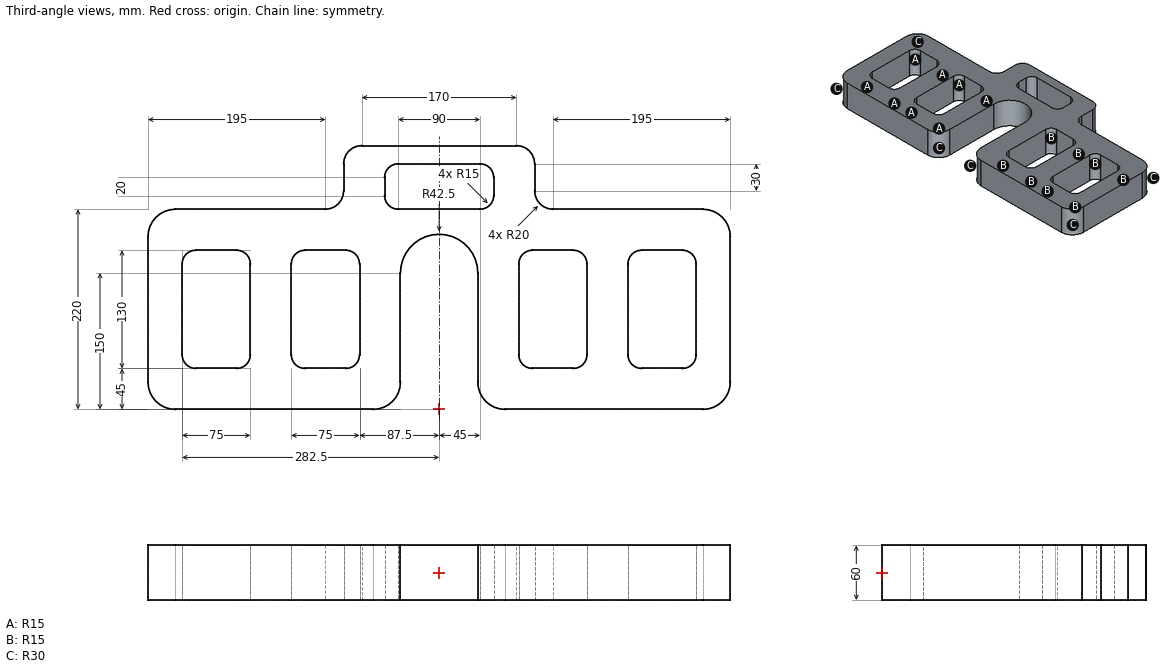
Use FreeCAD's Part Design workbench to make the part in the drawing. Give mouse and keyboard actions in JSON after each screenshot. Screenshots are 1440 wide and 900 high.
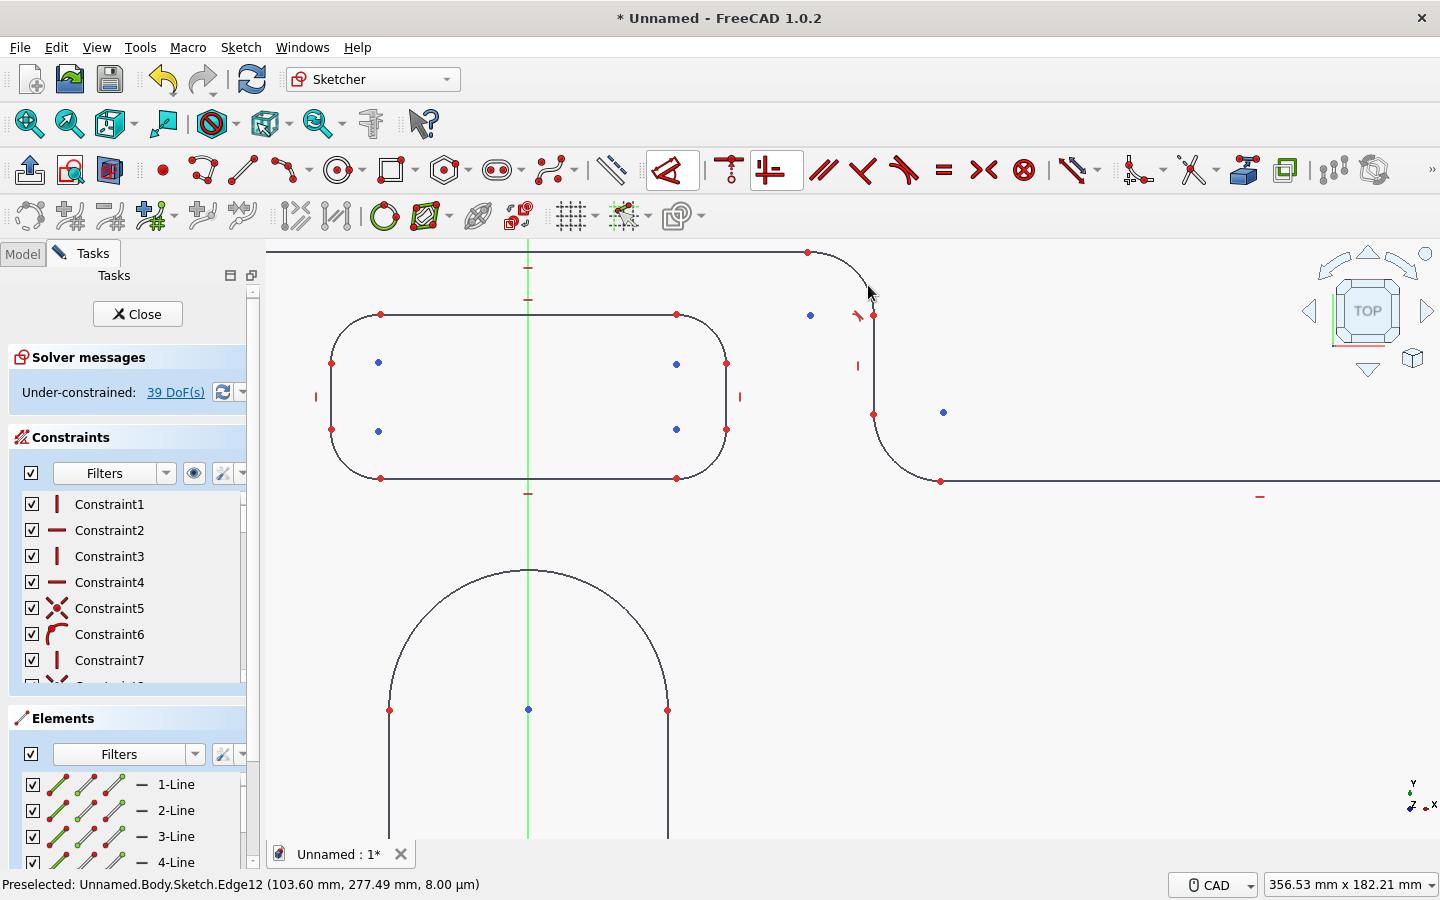
{"action": "left_click", "coordinate": [874, 385]}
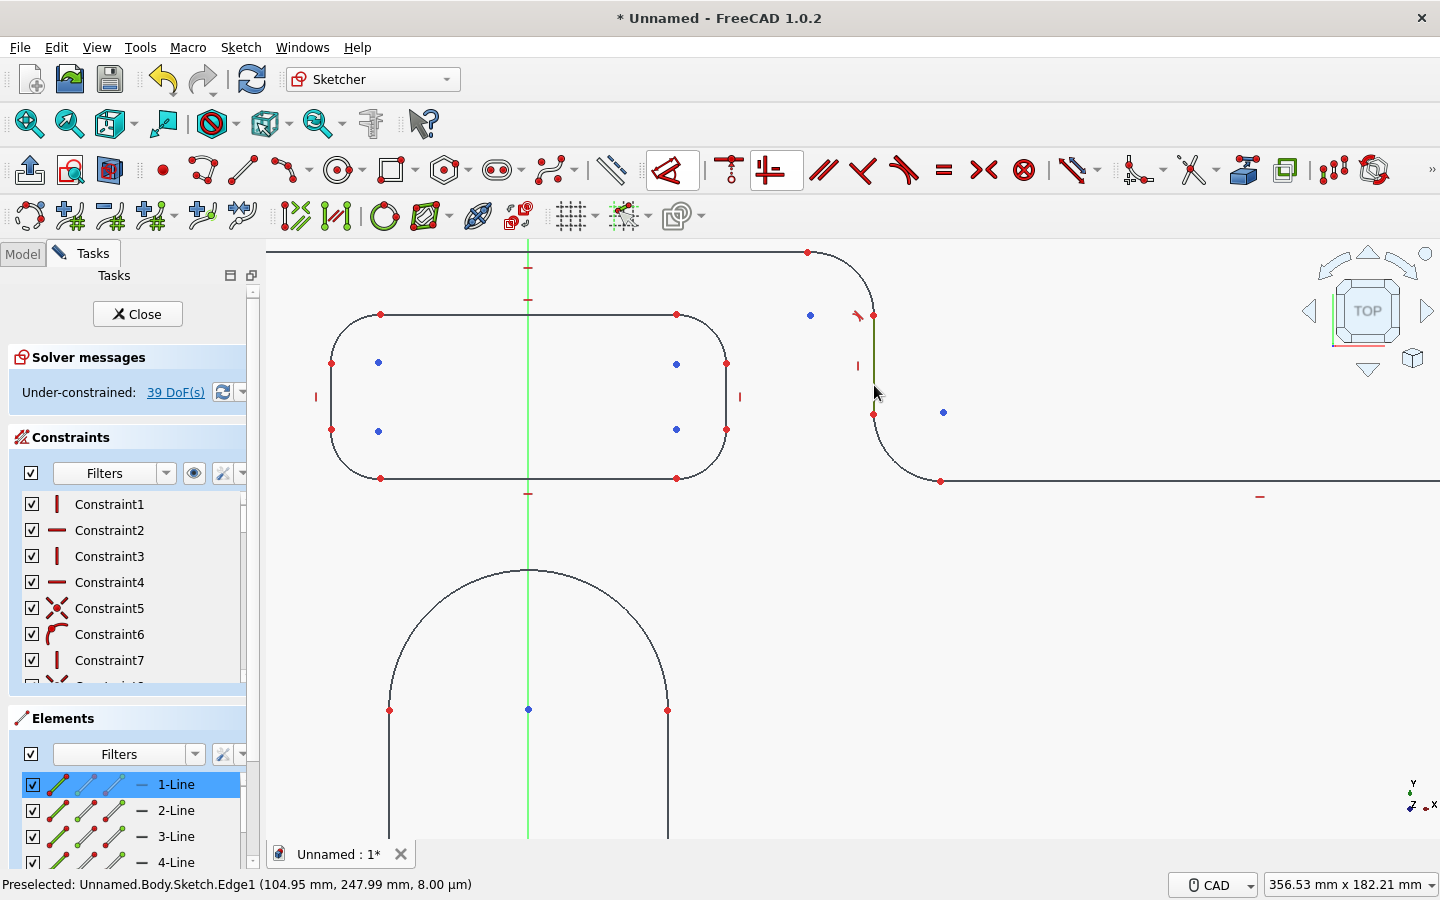
{"action": "left_click", "coordinate": [882, 445]}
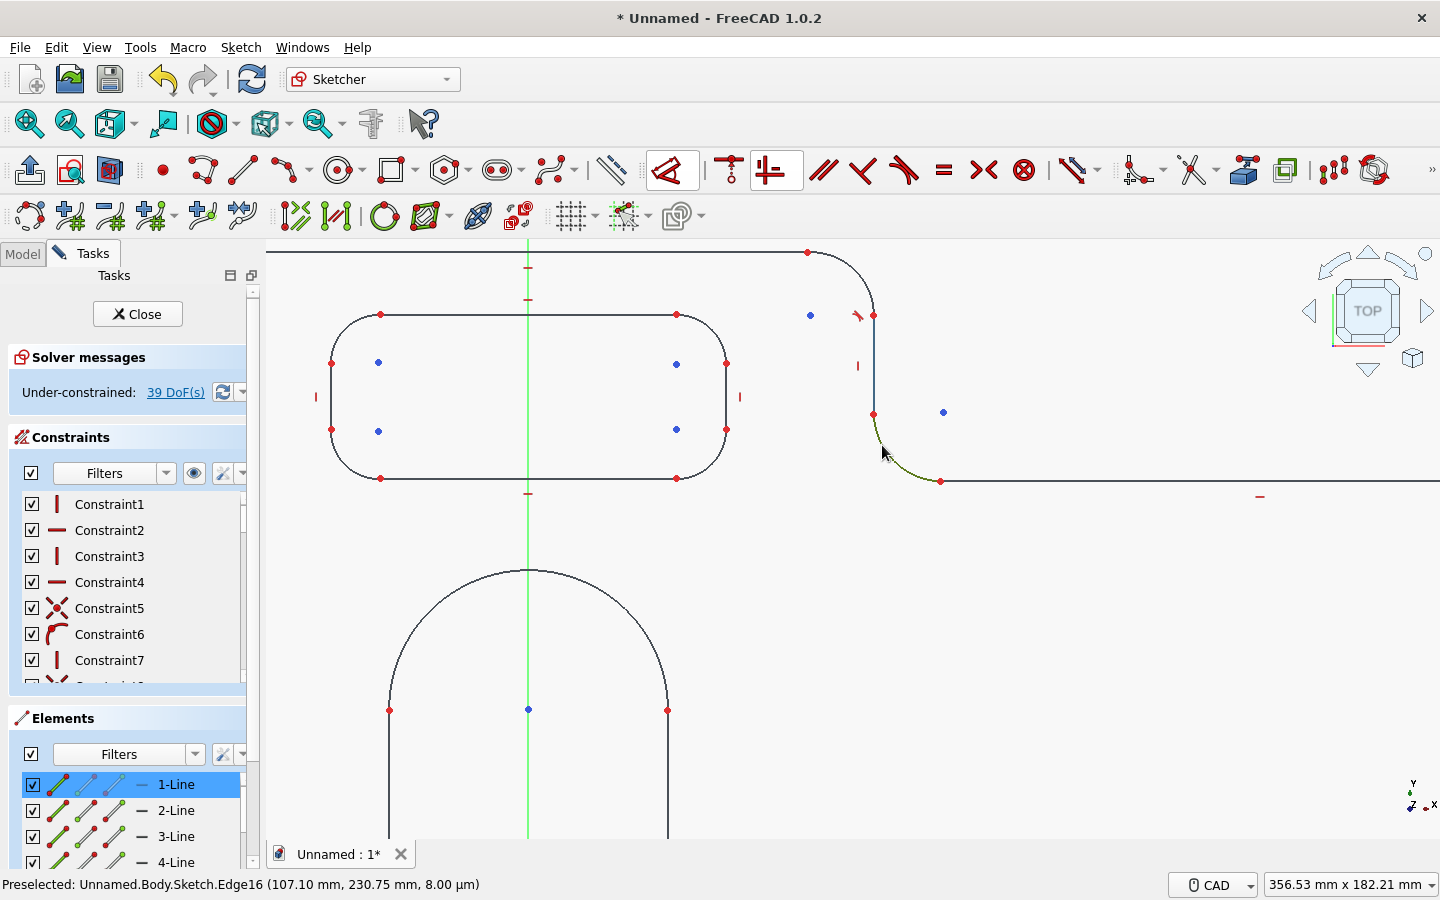
{"action": "left_click", "coordinate": [904, 170]}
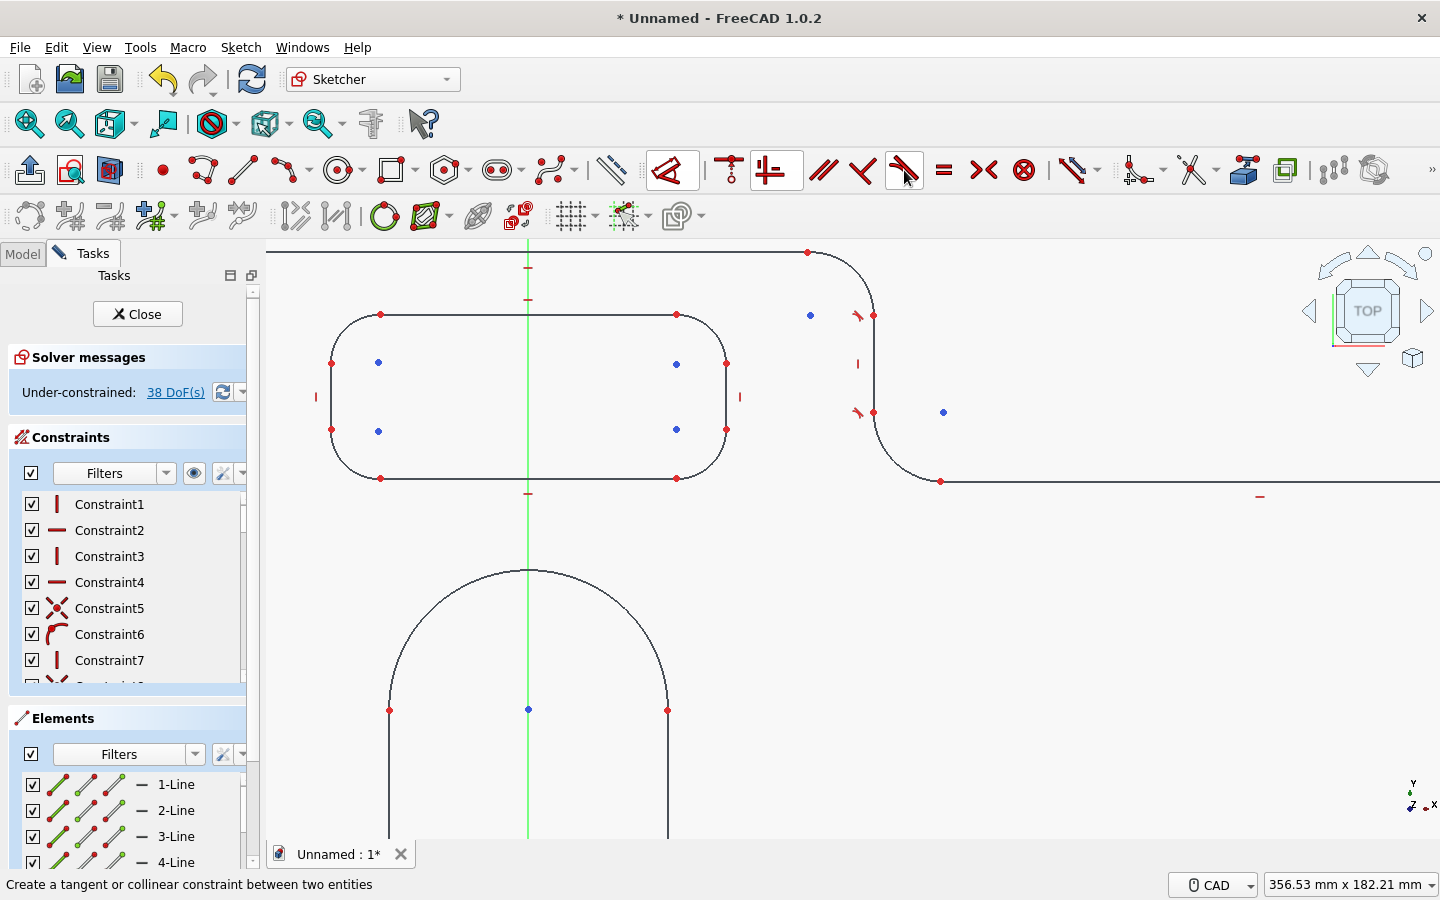
{"action": "scroll", "coordinate": [895, 459], "scroll_direction": "down", "scroll_amount": 6}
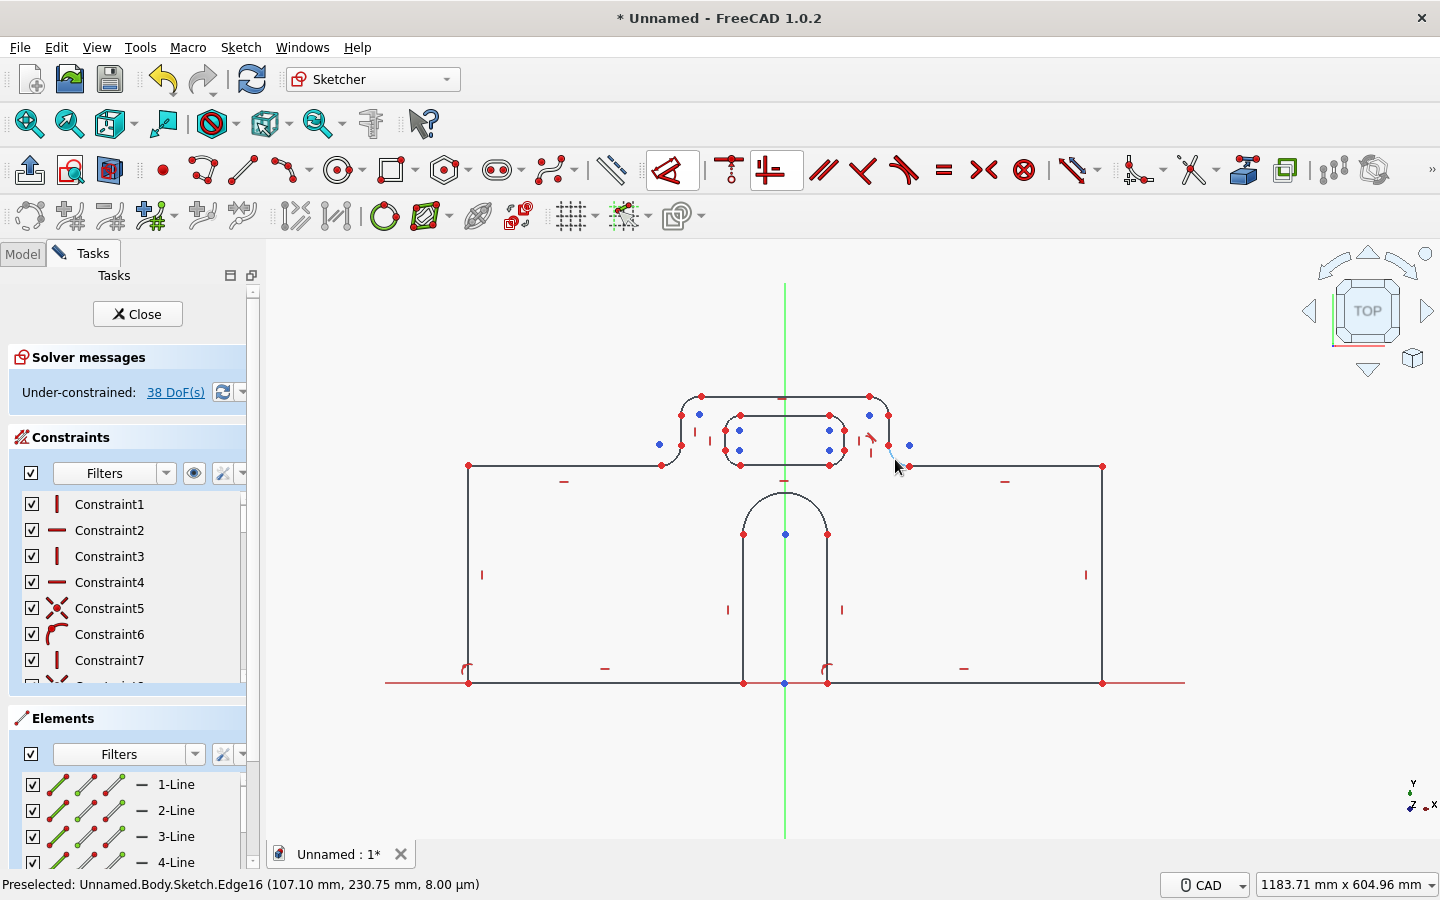
{"action": "left_click", "coordinate": [819, 397]}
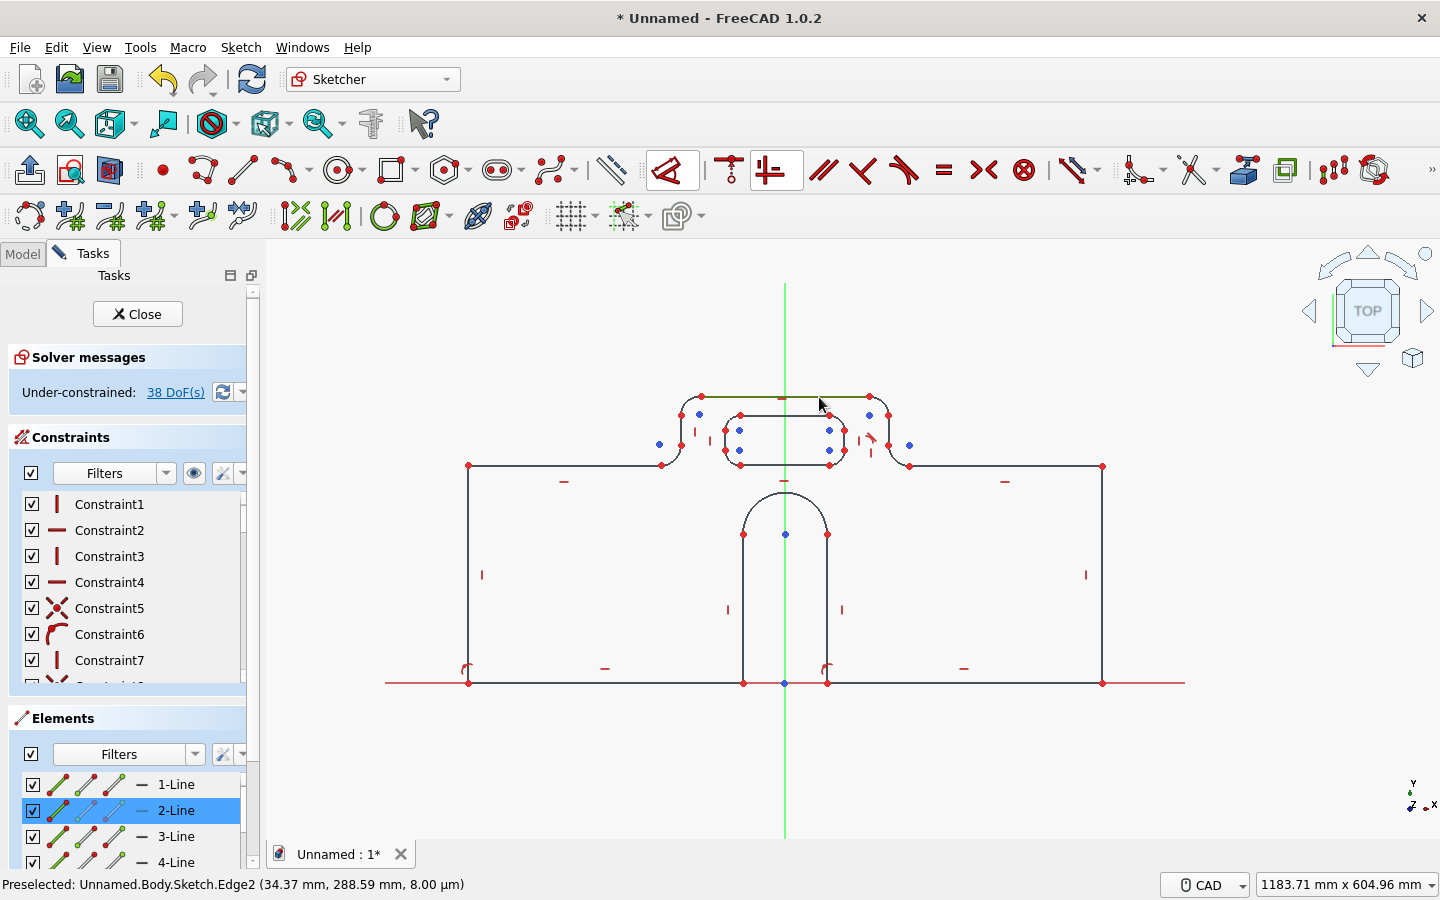
{"action": "scroll", "coordinate": [887, 407], "scroll_direction": "up", "scroll_amount": 3}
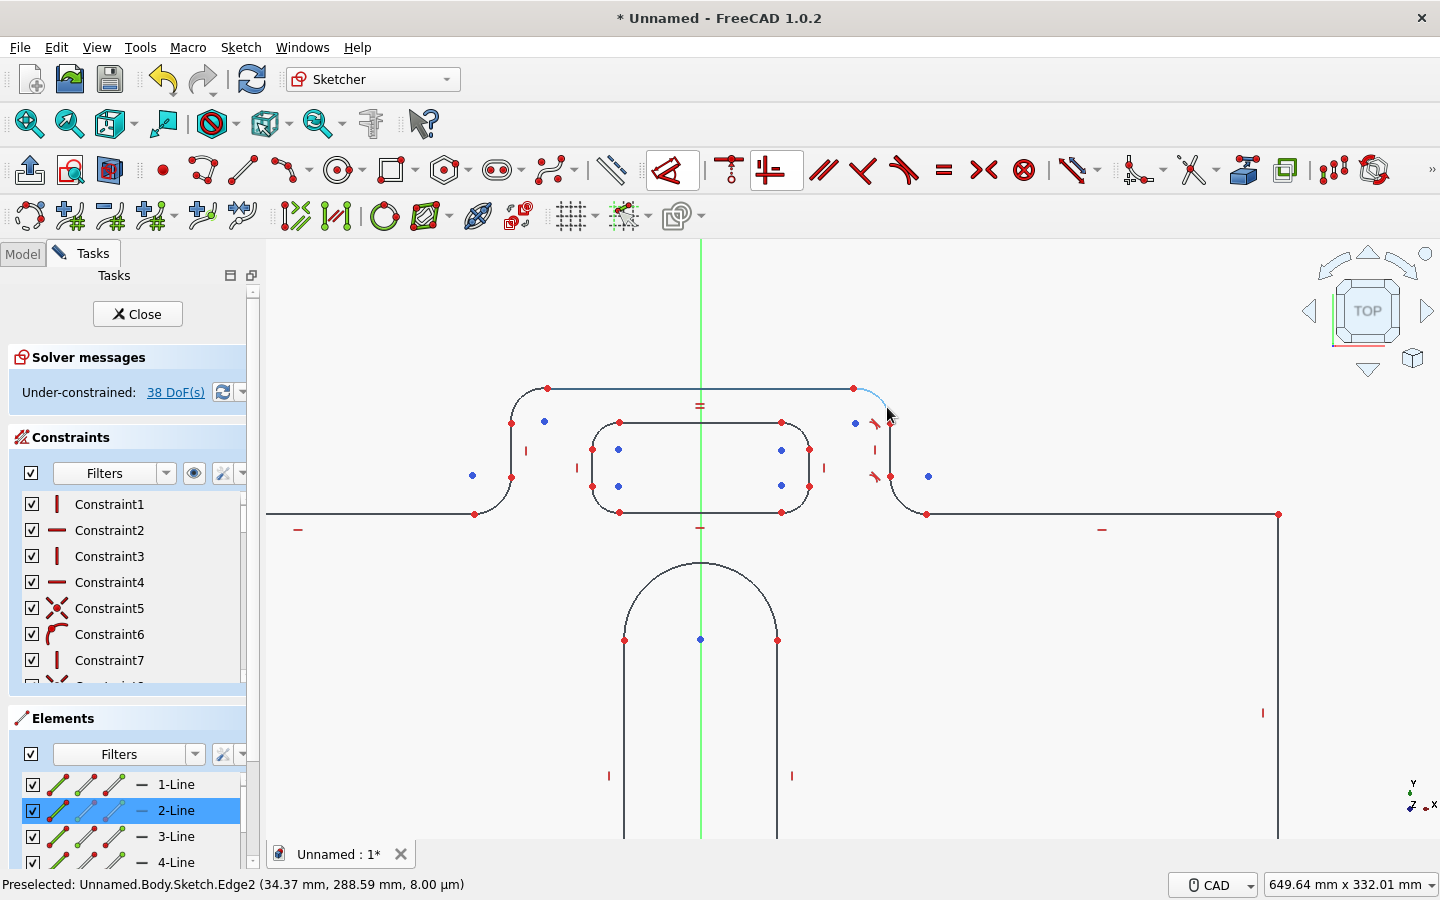
{"action": "left_click", "coordinate": [886, 407]}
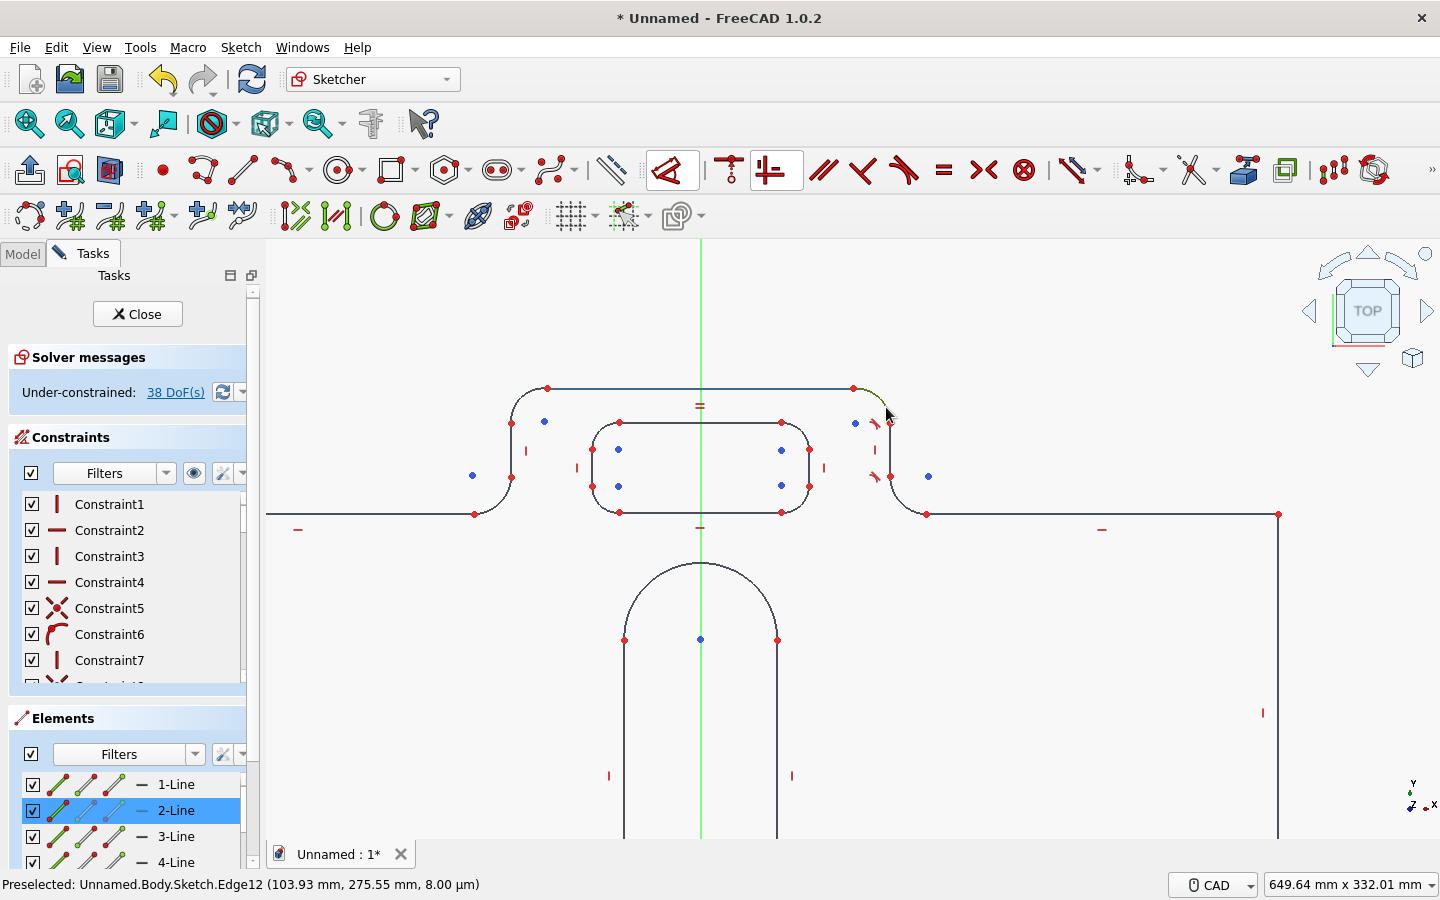
{"action": "key", "text": "t"}